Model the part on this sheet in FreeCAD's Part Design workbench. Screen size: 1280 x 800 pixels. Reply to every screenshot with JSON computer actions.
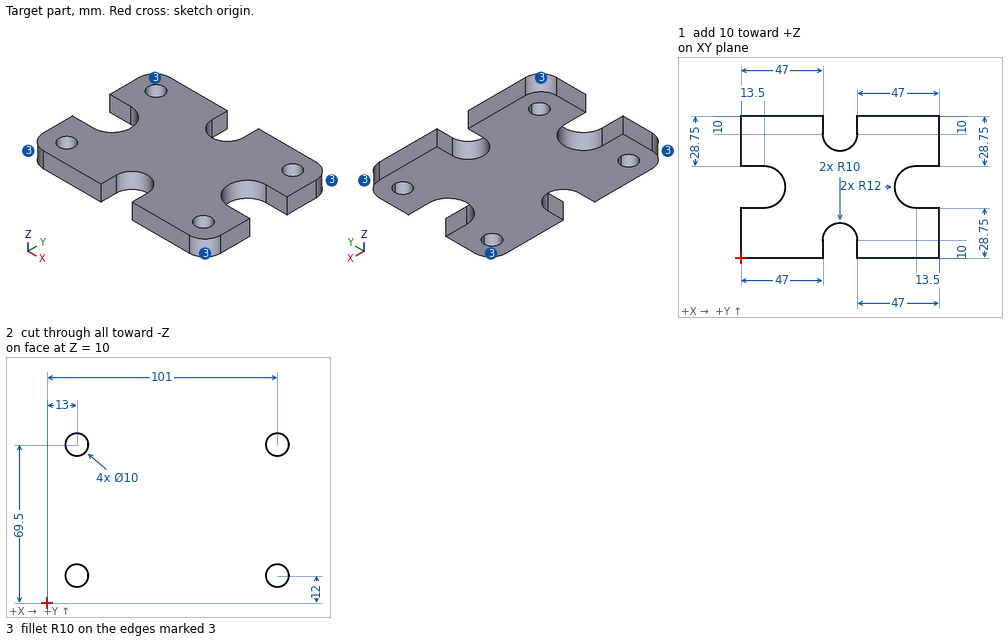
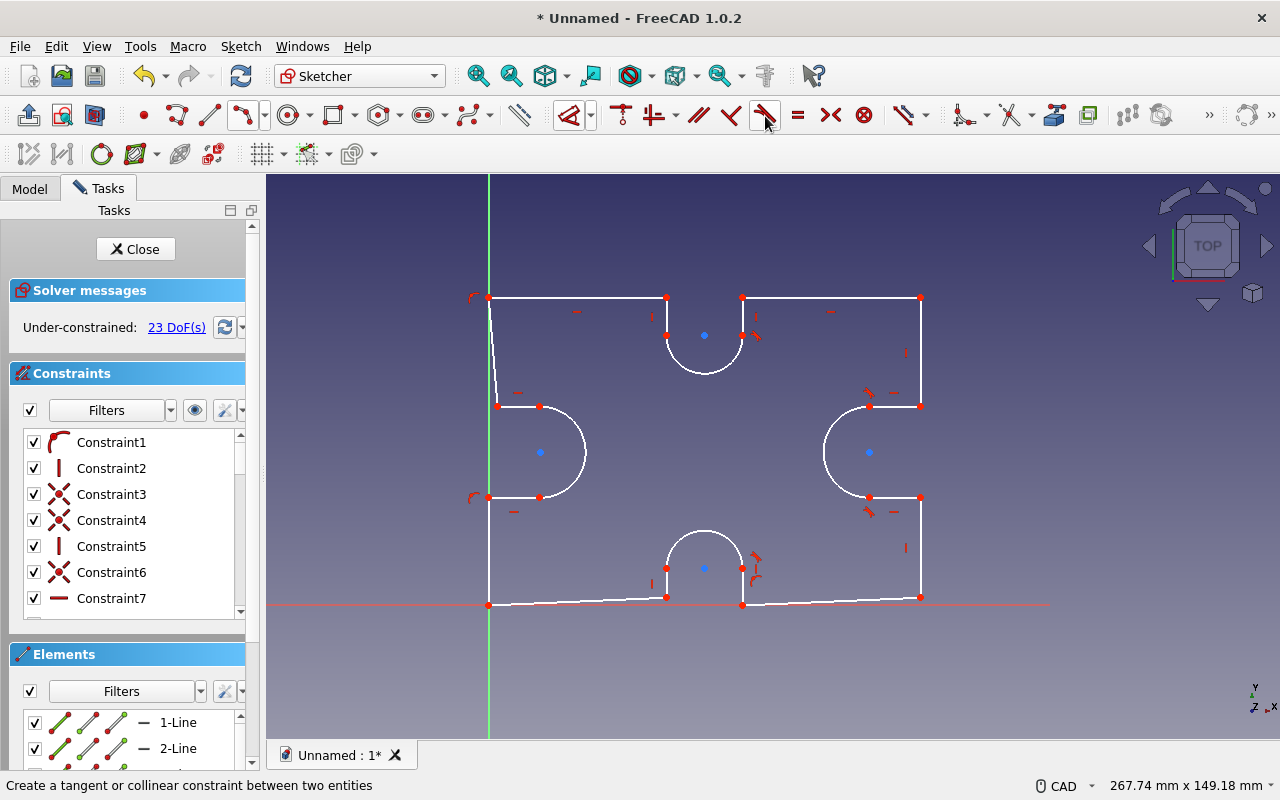
{"action": "left_click", "coordinate": [667, 324]}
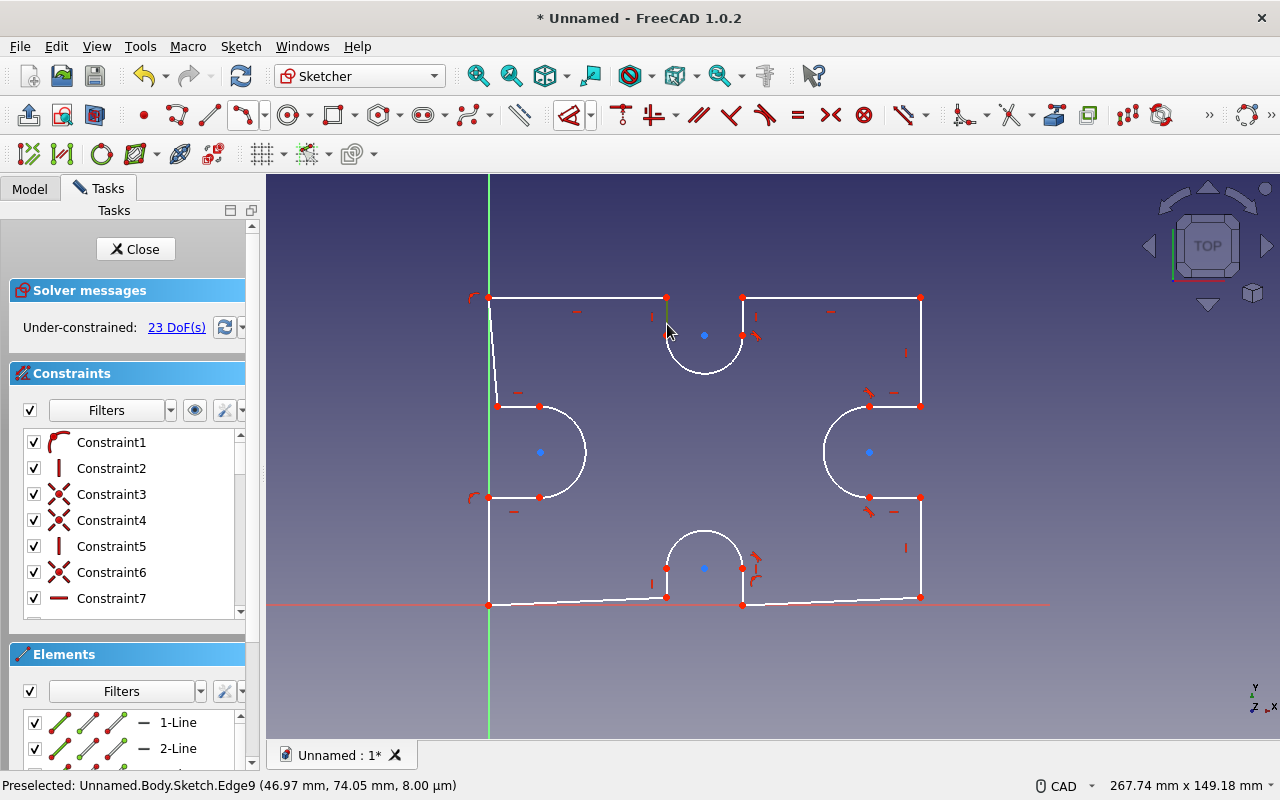
{"action": "left_click", "coordinate": [682, 366]}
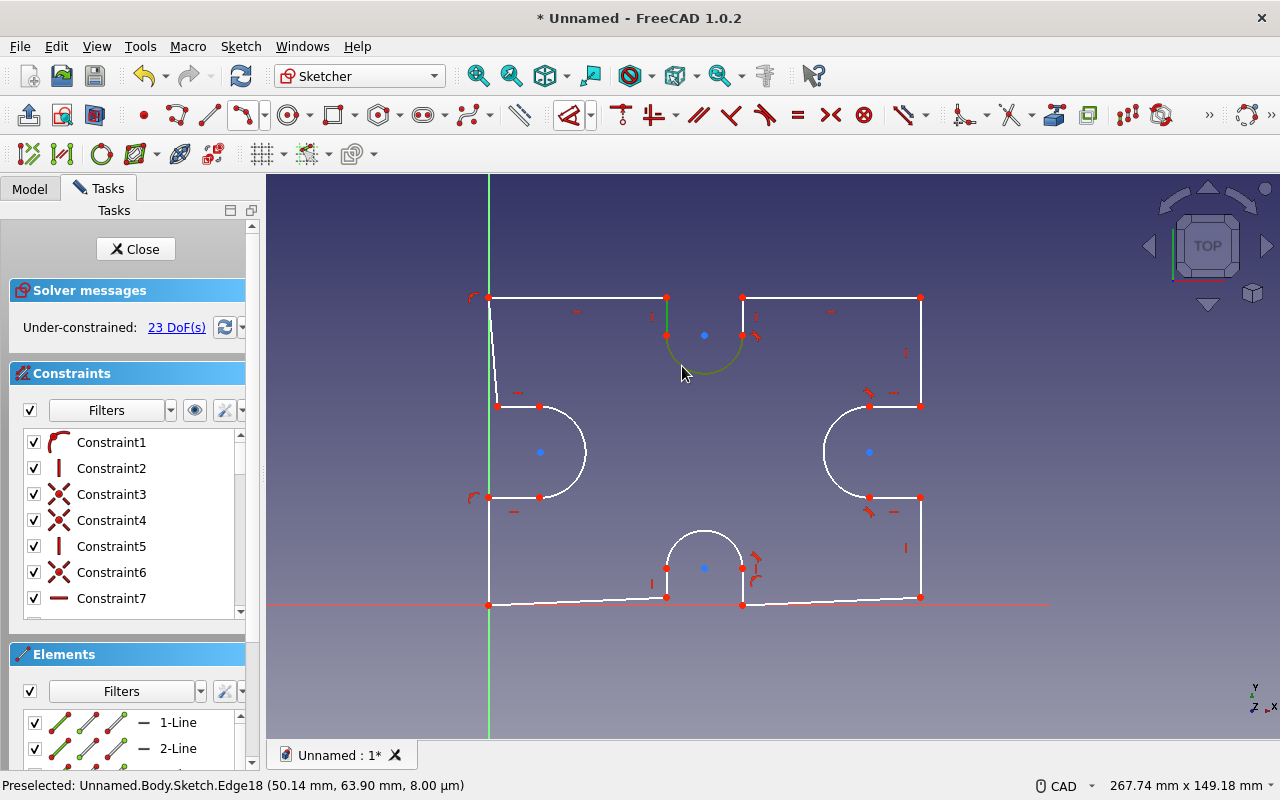
{"action": "left_click", "coordinate": [765, 116]}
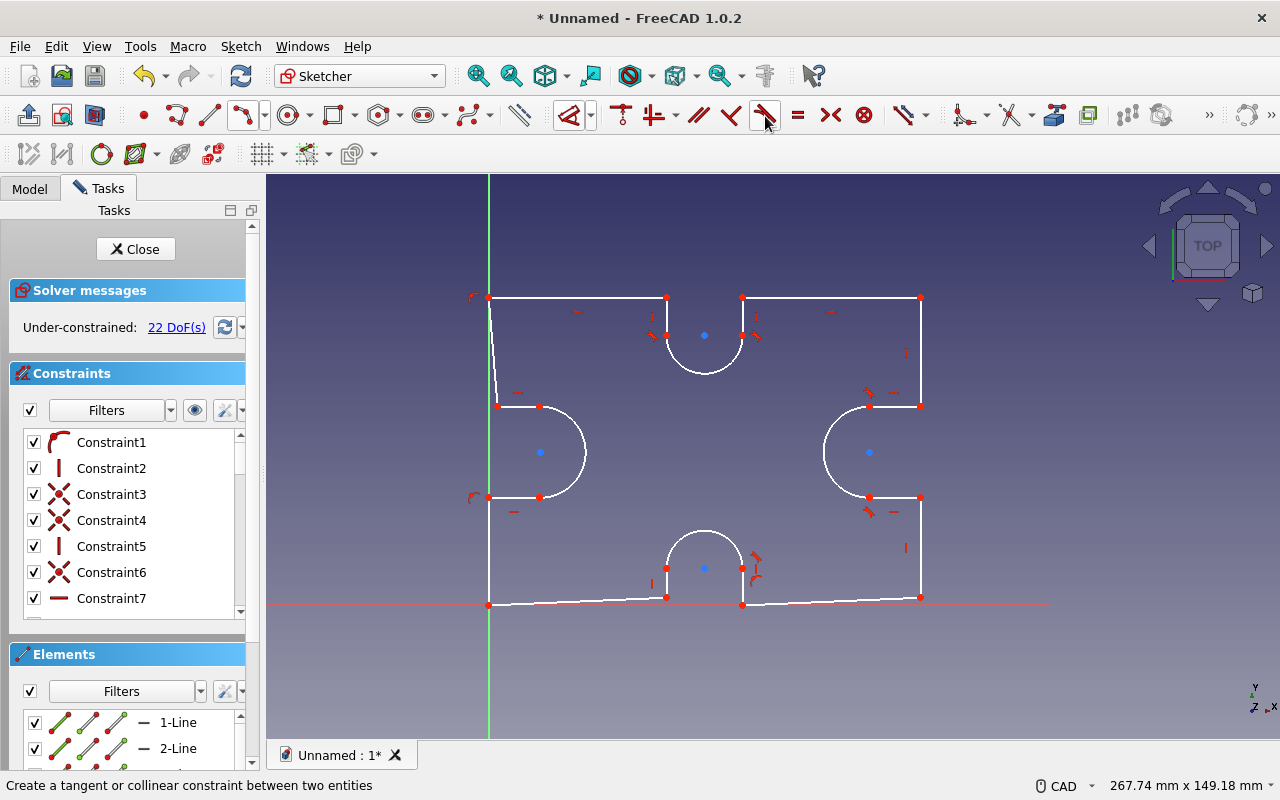
{"action": "left_click", "coordinate": [510, 407]}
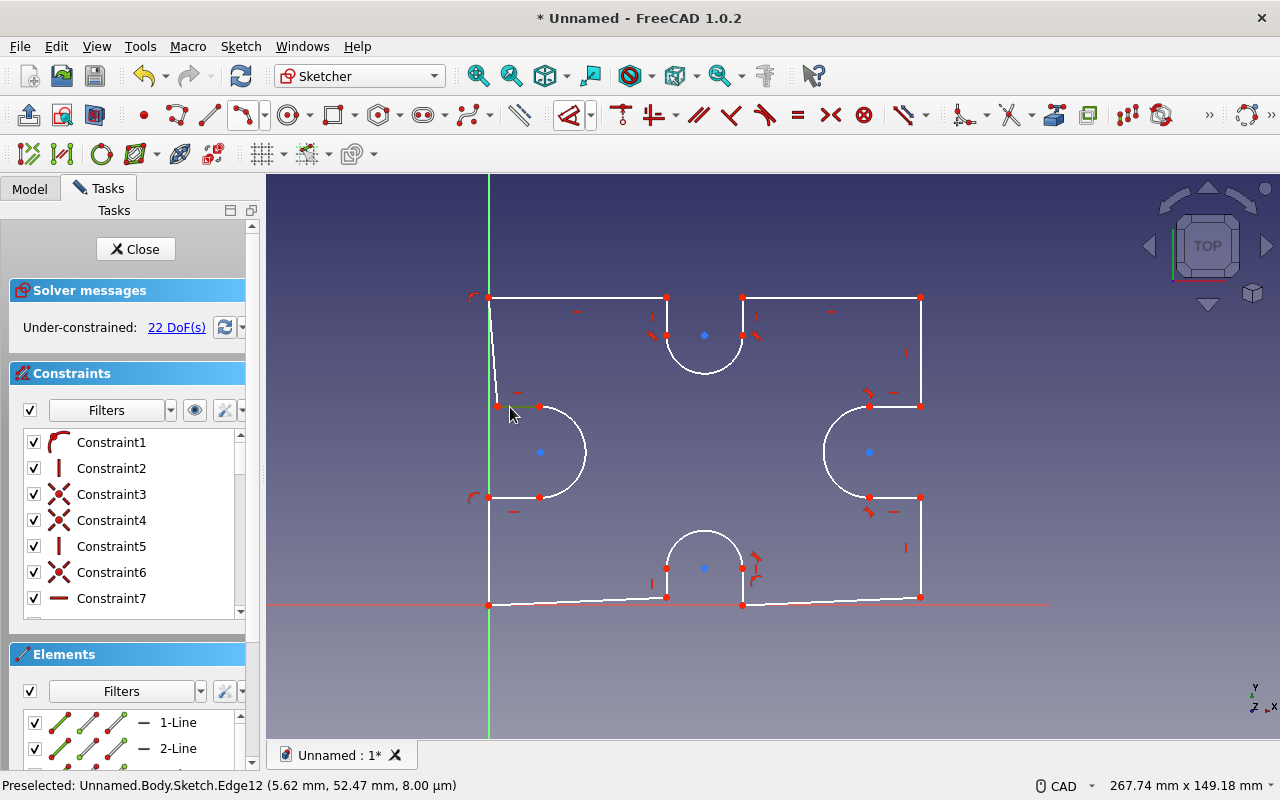
{"action": "left_click", "coordinate": [577, 479]}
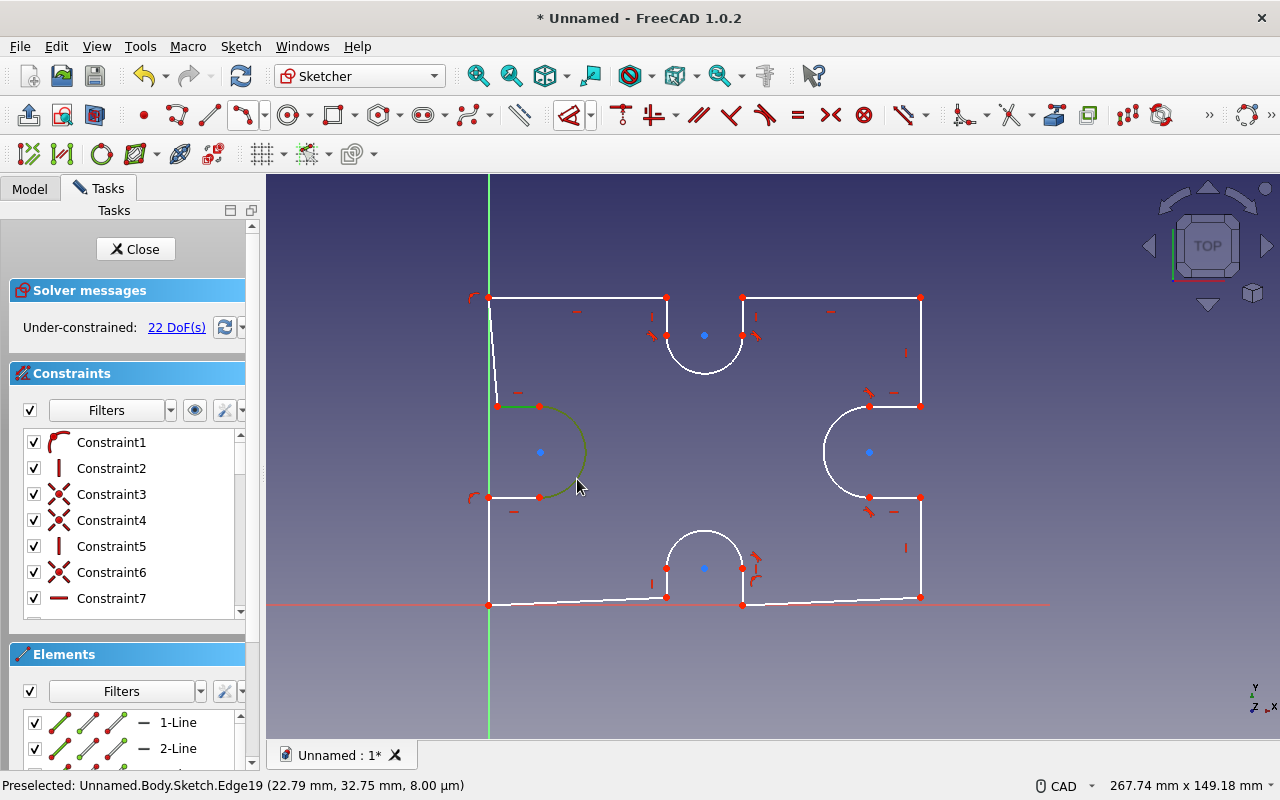
{"action": "left_click", "coordinate": [765, 116]}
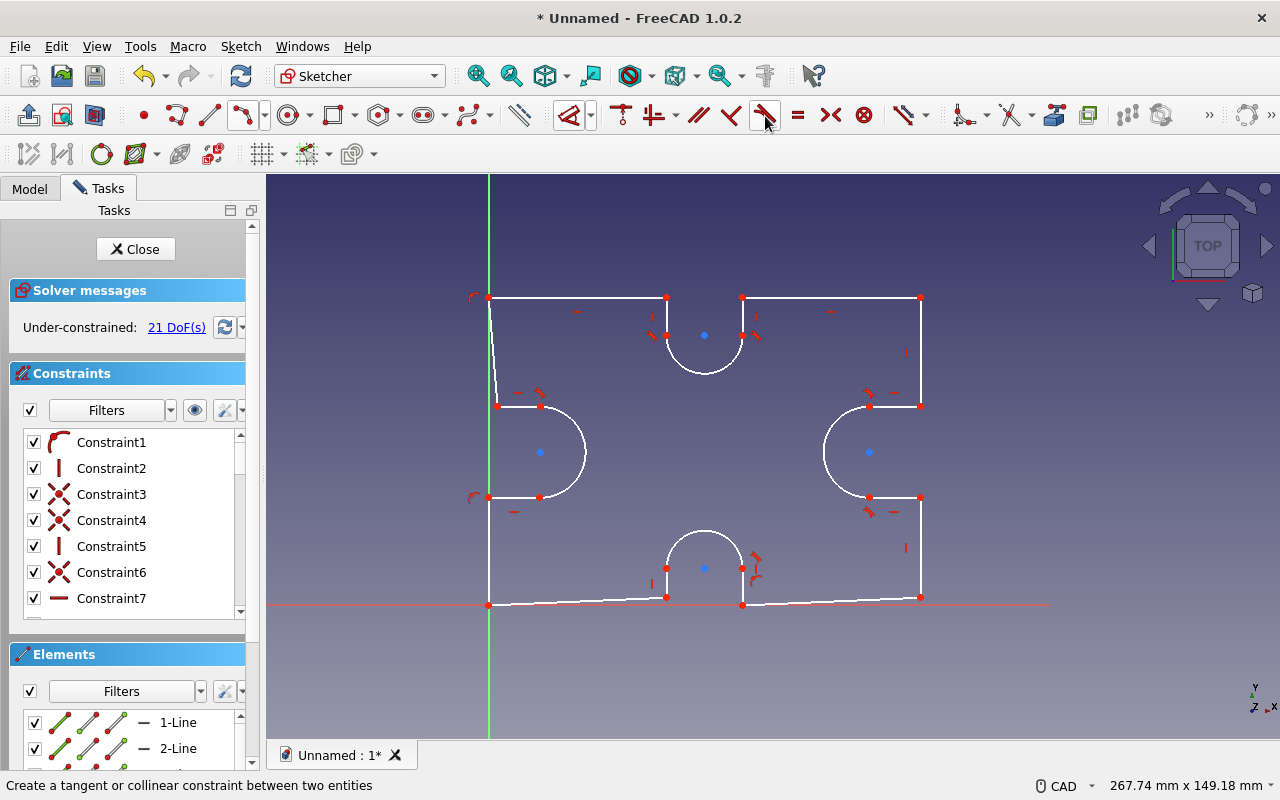
{"action": "left_click", "coordinate": [524, 498]}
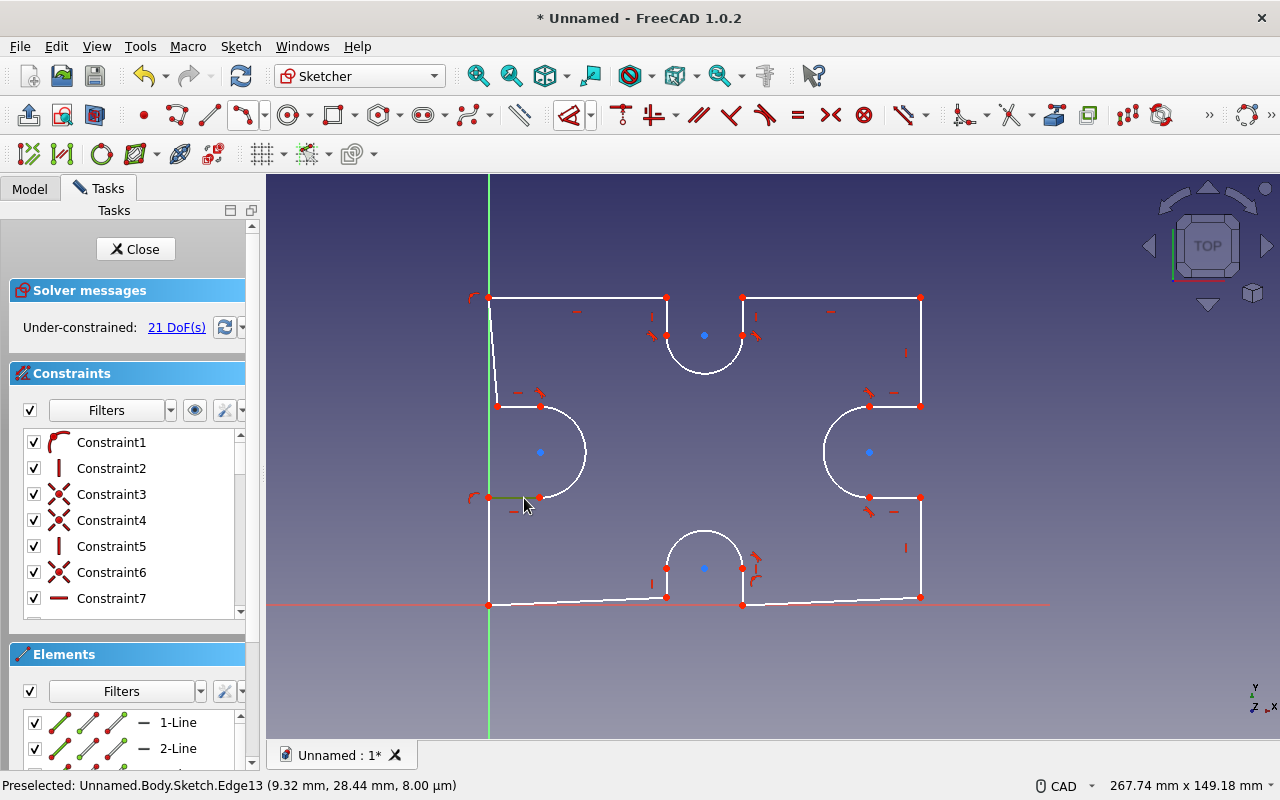
{"action": "left_click", "coordinate": [577, 479]}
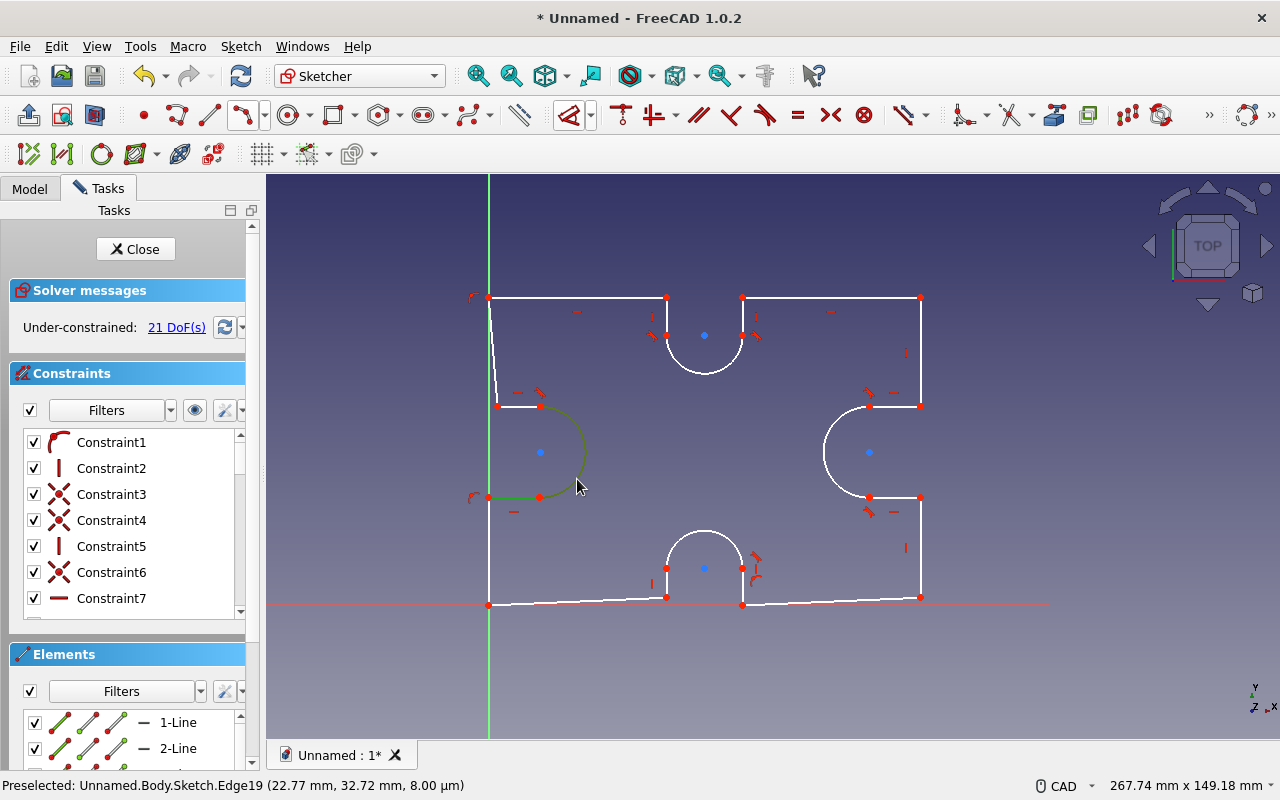
{"action": "left_click", "coordinate": [765, 116]}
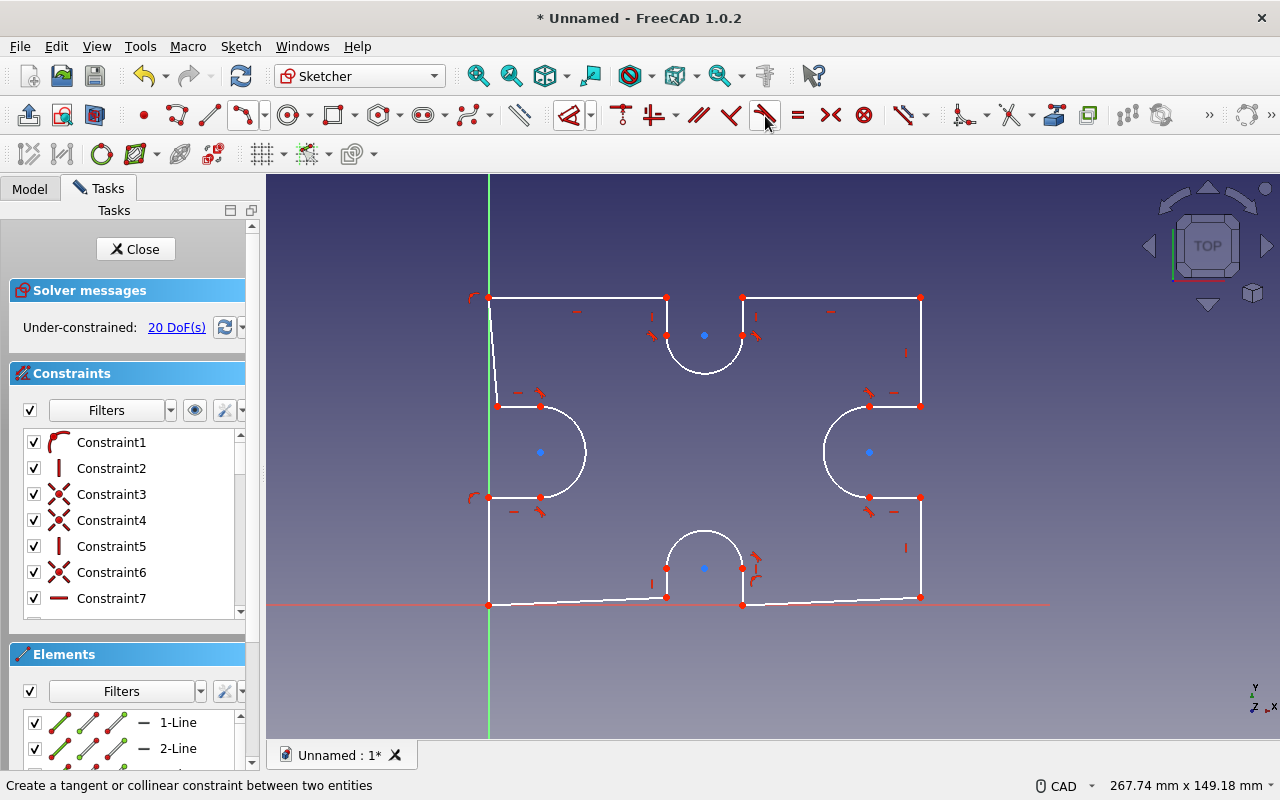
{"action": "left_click", "coordinate": [667, 586]}